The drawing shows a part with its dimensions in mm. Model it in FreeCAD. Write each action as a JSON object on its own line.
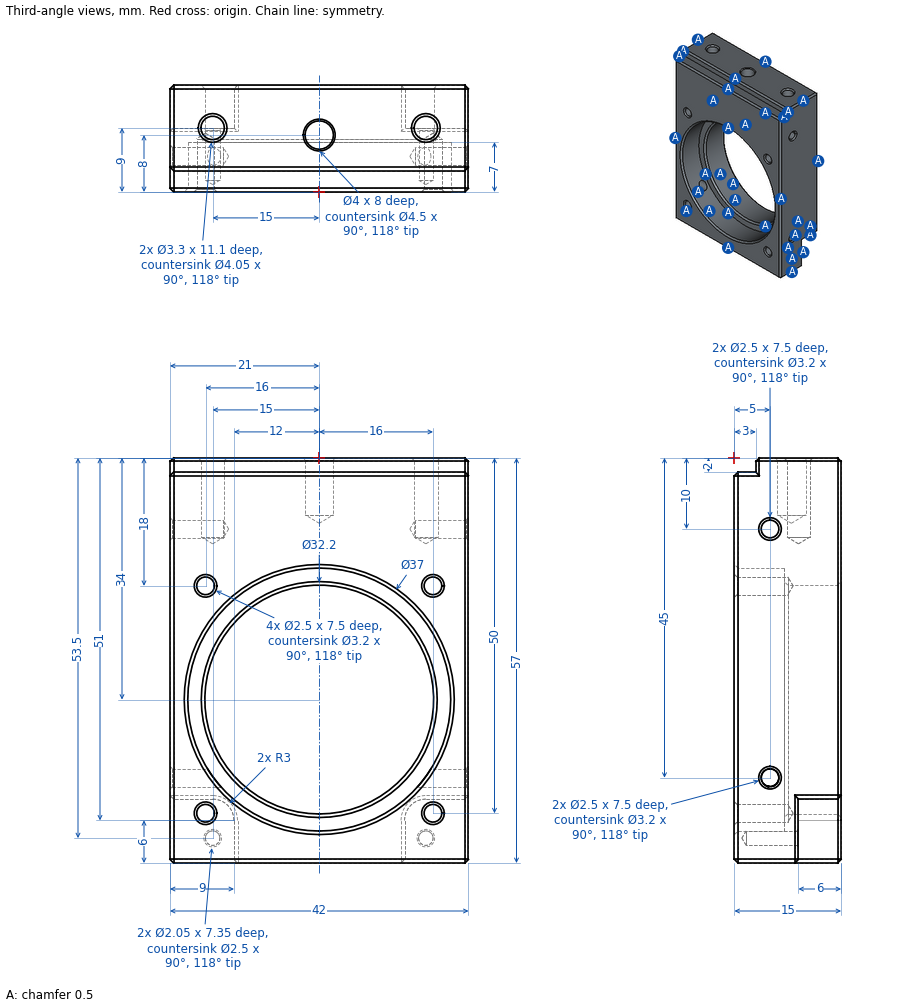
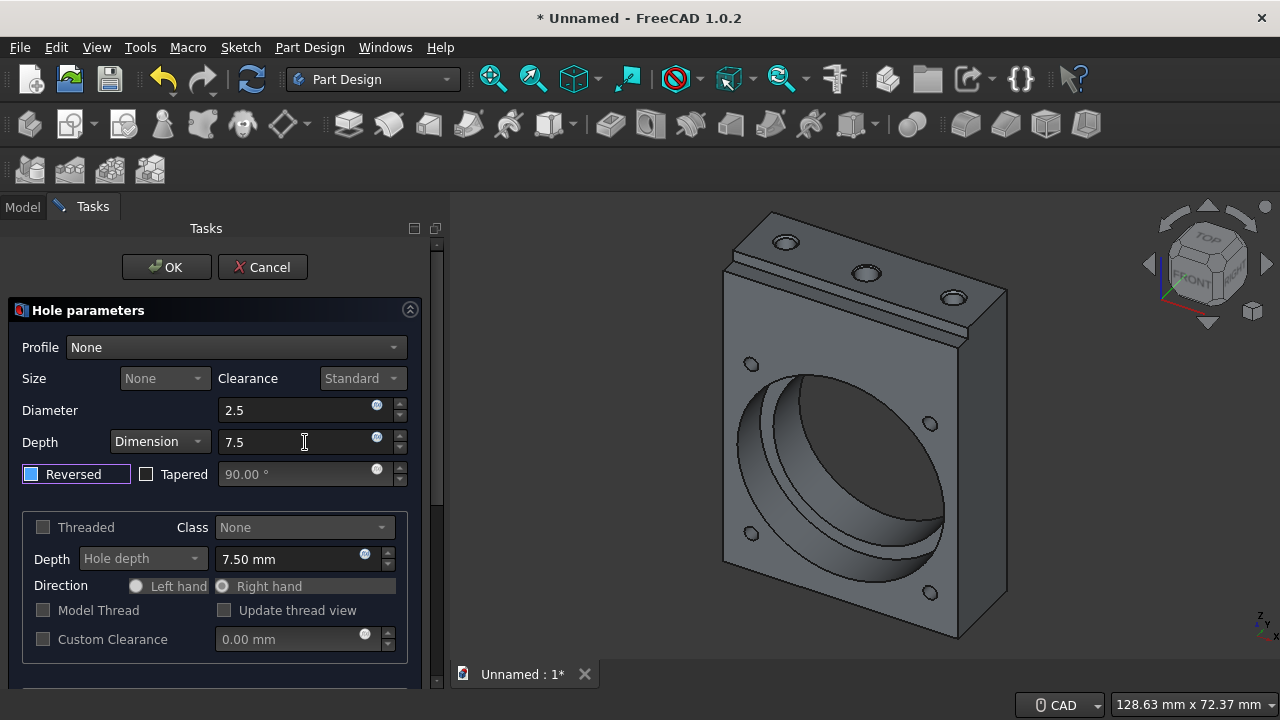
{"action": "scroll", "coordinate": [437, 463], "scroll_direction": "down", "scroll_amount": 2}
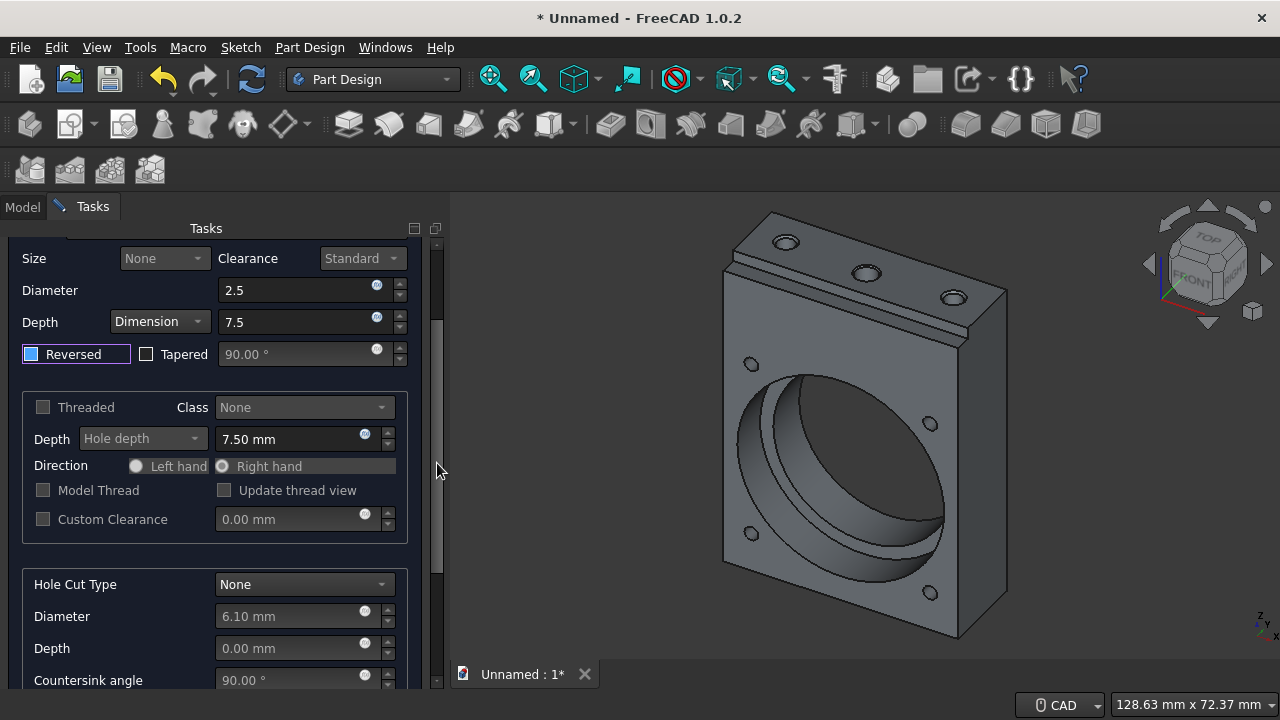
{"action": "left_click", "coordinate": [306, 584]}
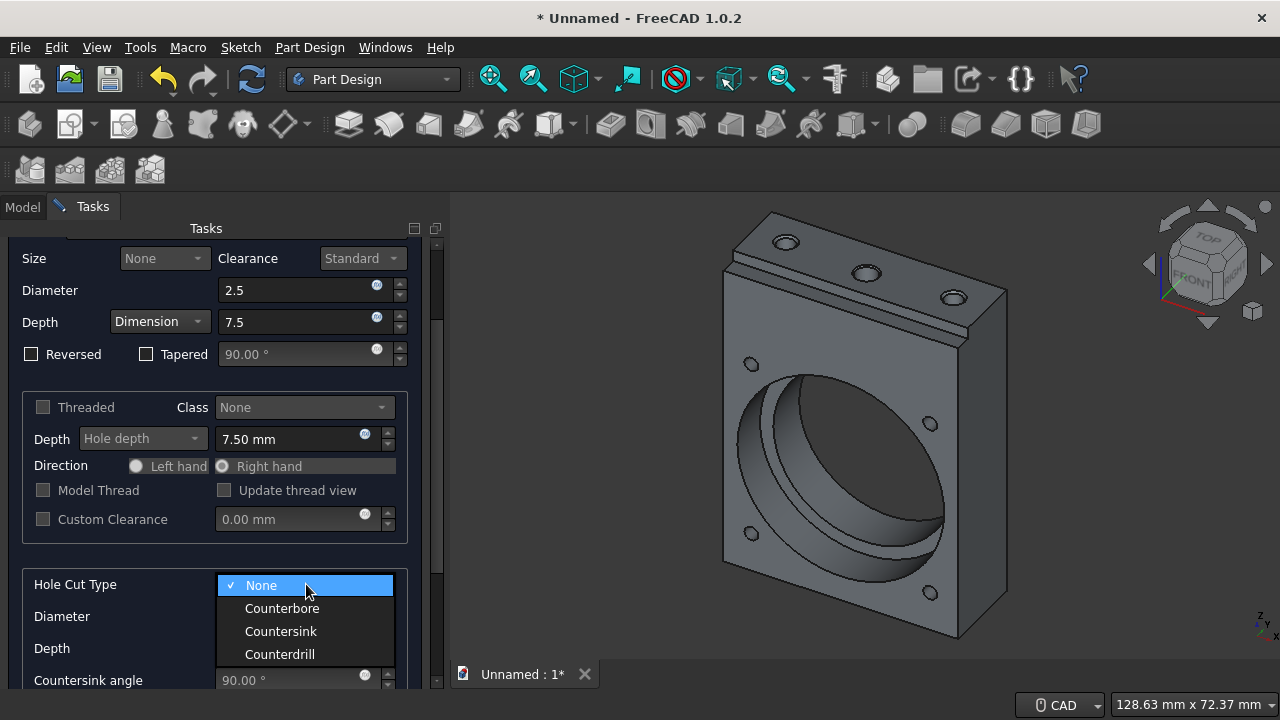
{"action": "left_click", "coordinate": [304, 632]}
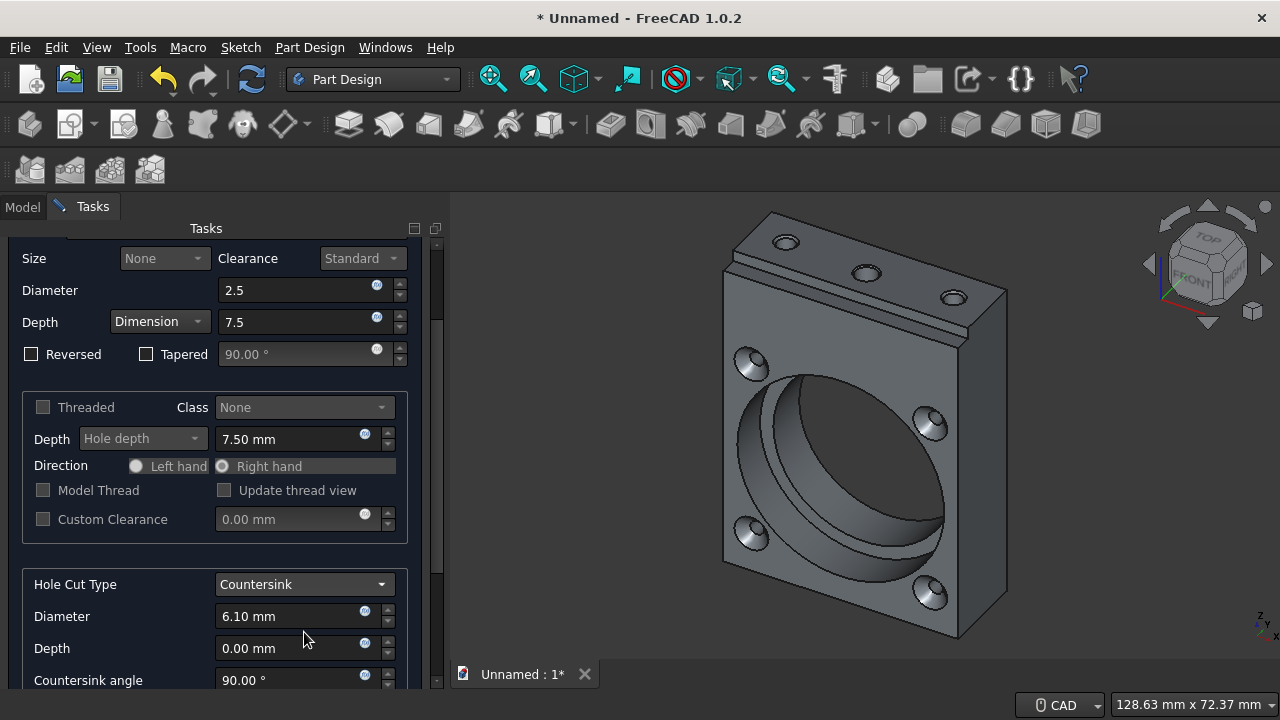
{"action": "triple_click", "coordinate": [298, 616]}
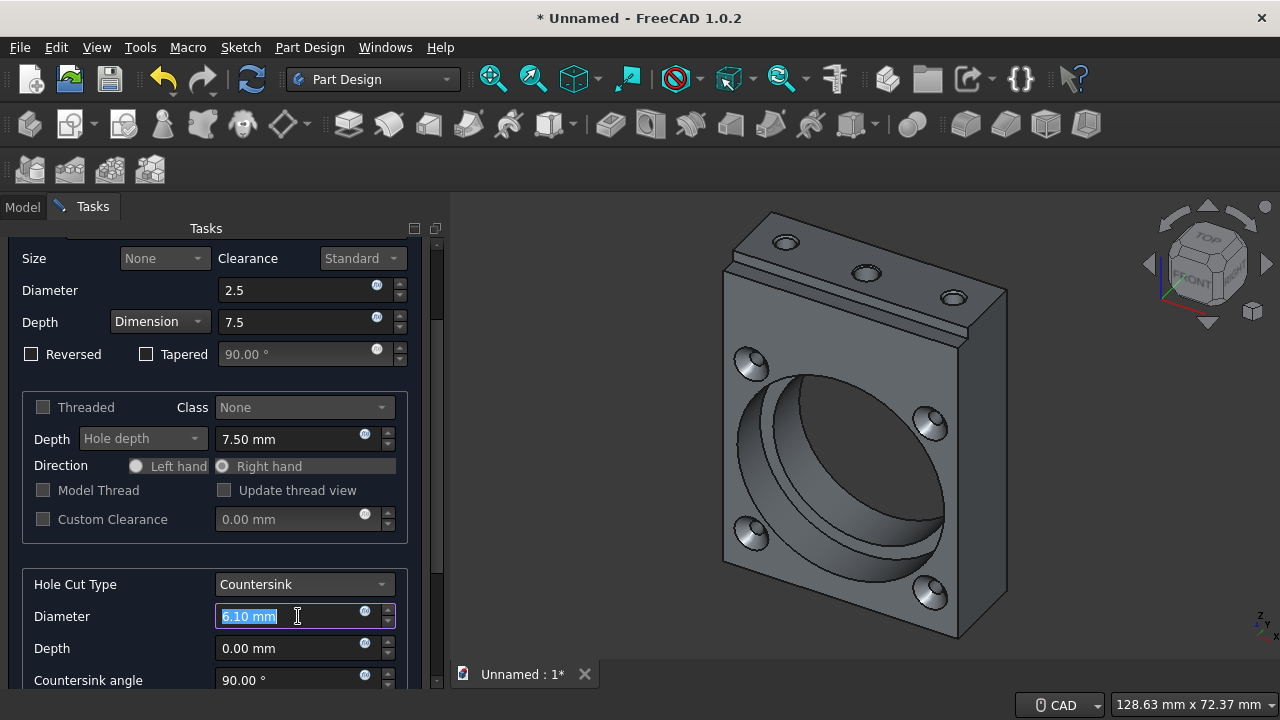
{"action": "type", "text": "3.2"}
{"action": "key", "text": "Tab"}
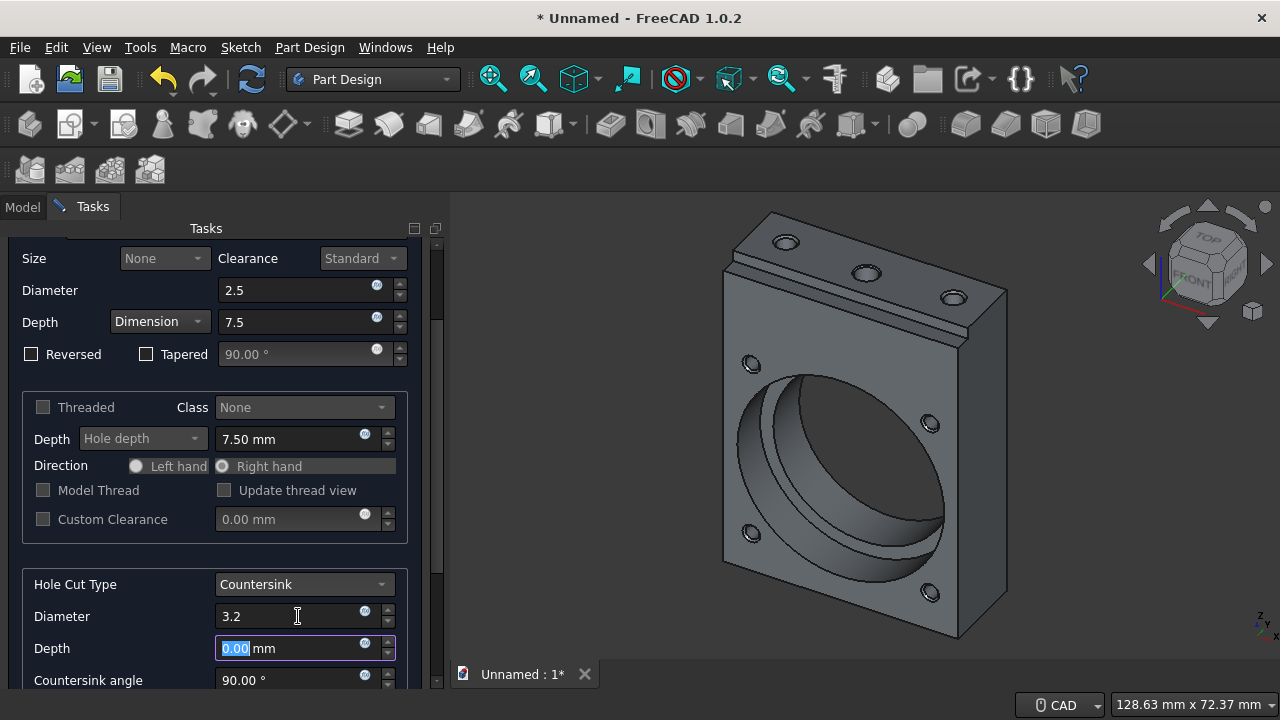
{"action": "scroll", "coordinate": [437, 463], "scroll_direction": "up", "scroll_amount": 3}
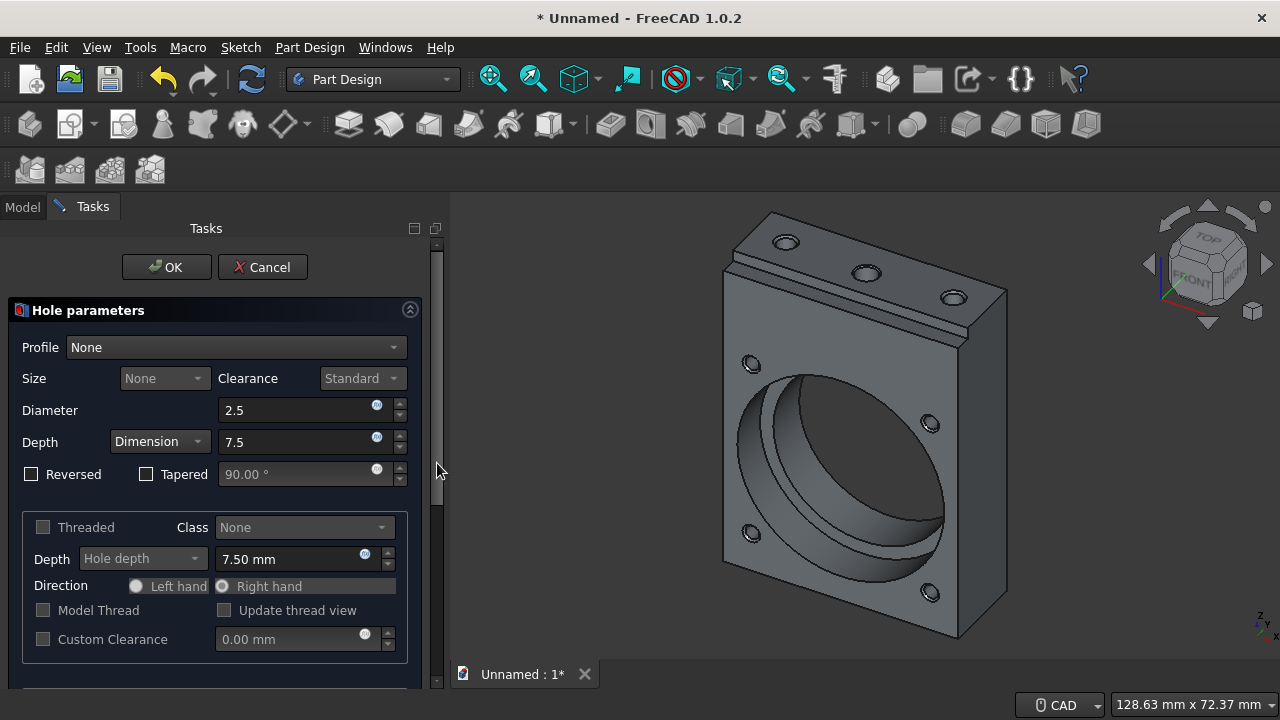
{"action": "left_click", "coordinate": [167, 267]}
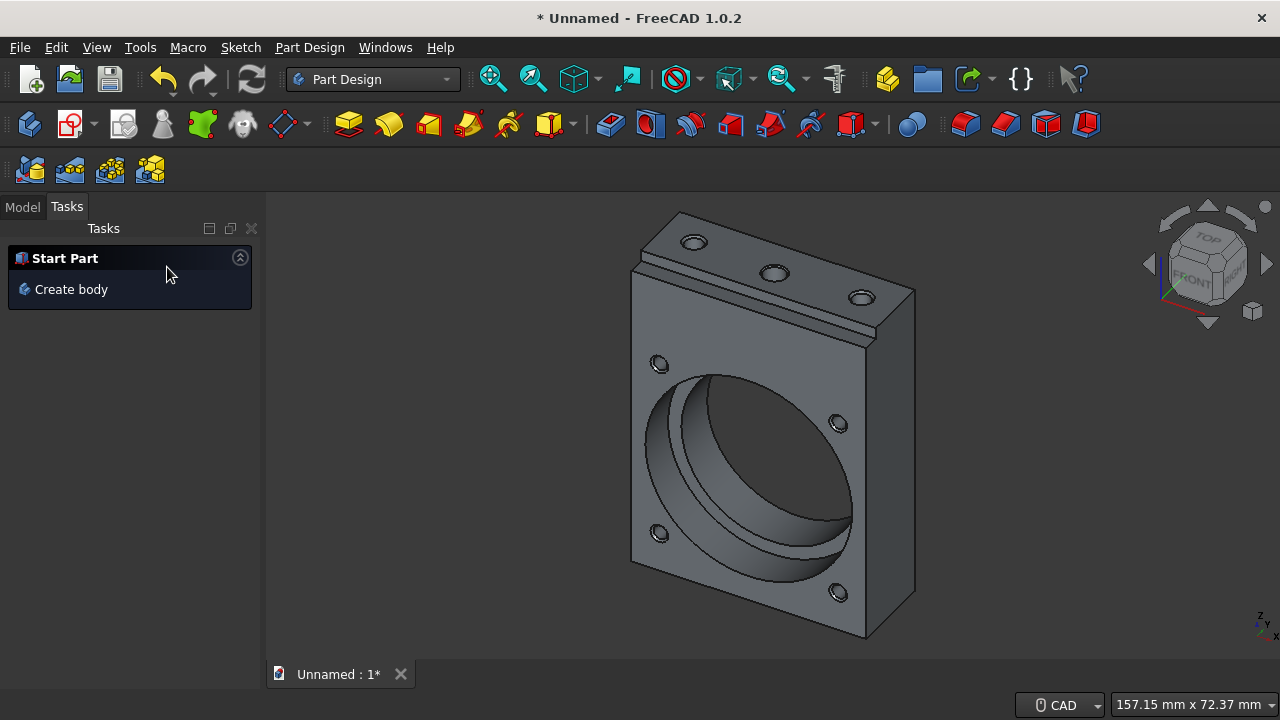
{"action": "key", "text": "4"}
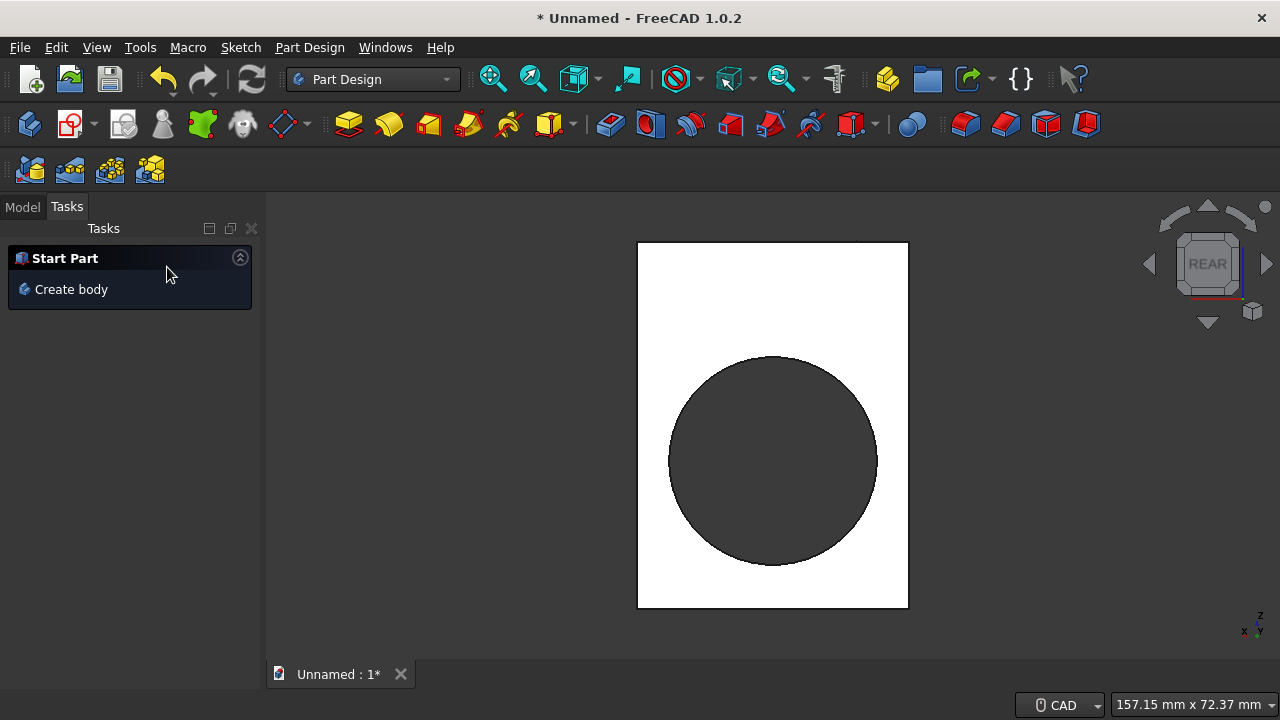
{"action": "left_click", "coordinate": [696, 319]}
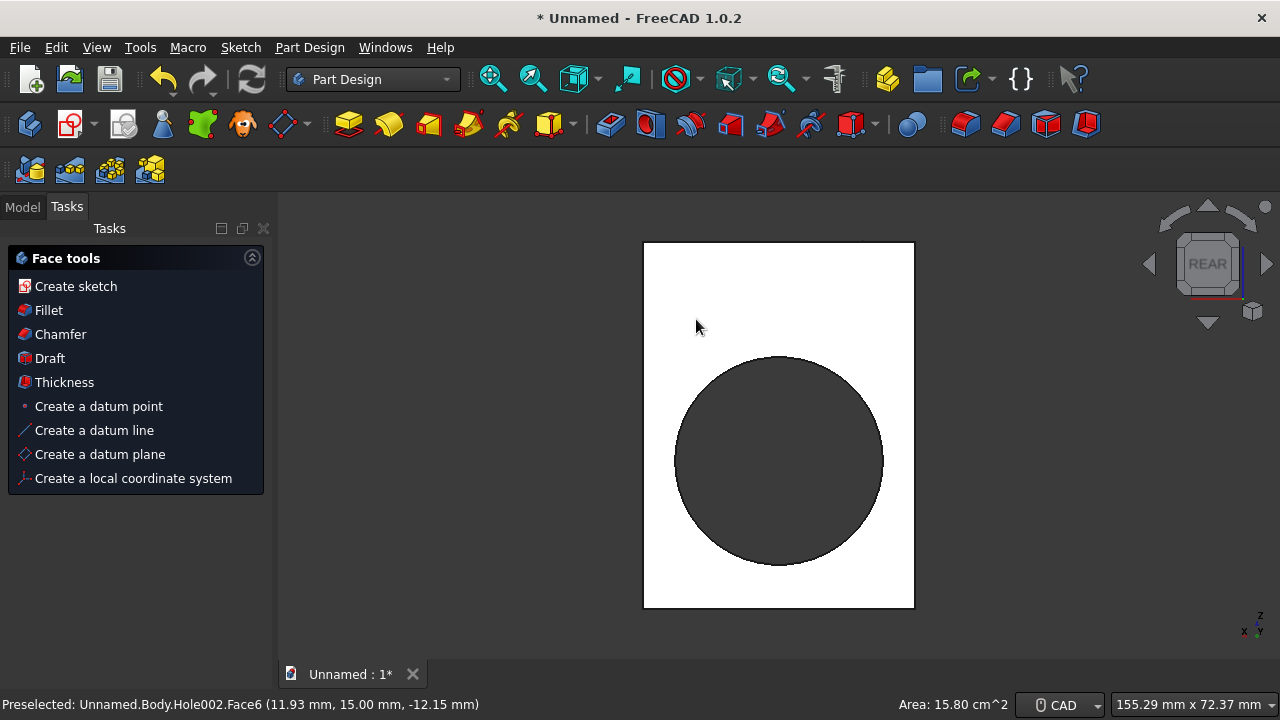
{"action": "left_click", "coordinate": [70, 124]}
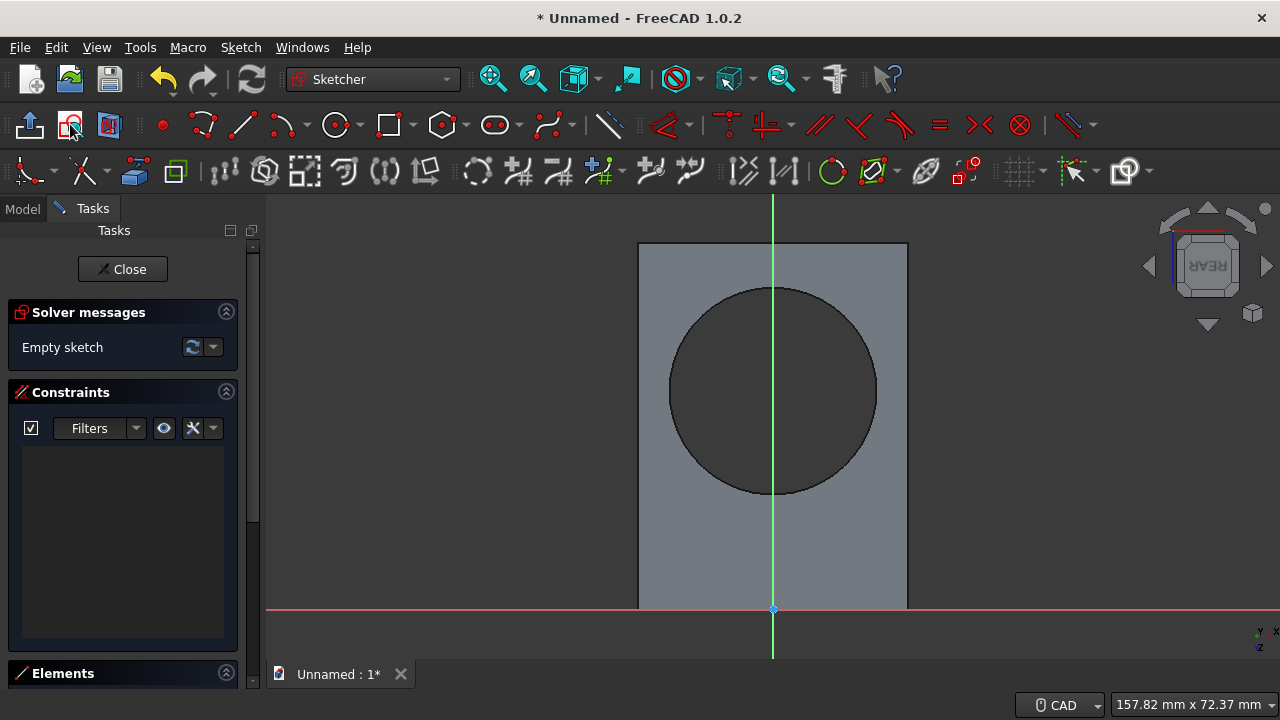
{"action": "scroll", "coordinate": [395, 426], "scroll_direction": "down", "scroll_amount": 1}